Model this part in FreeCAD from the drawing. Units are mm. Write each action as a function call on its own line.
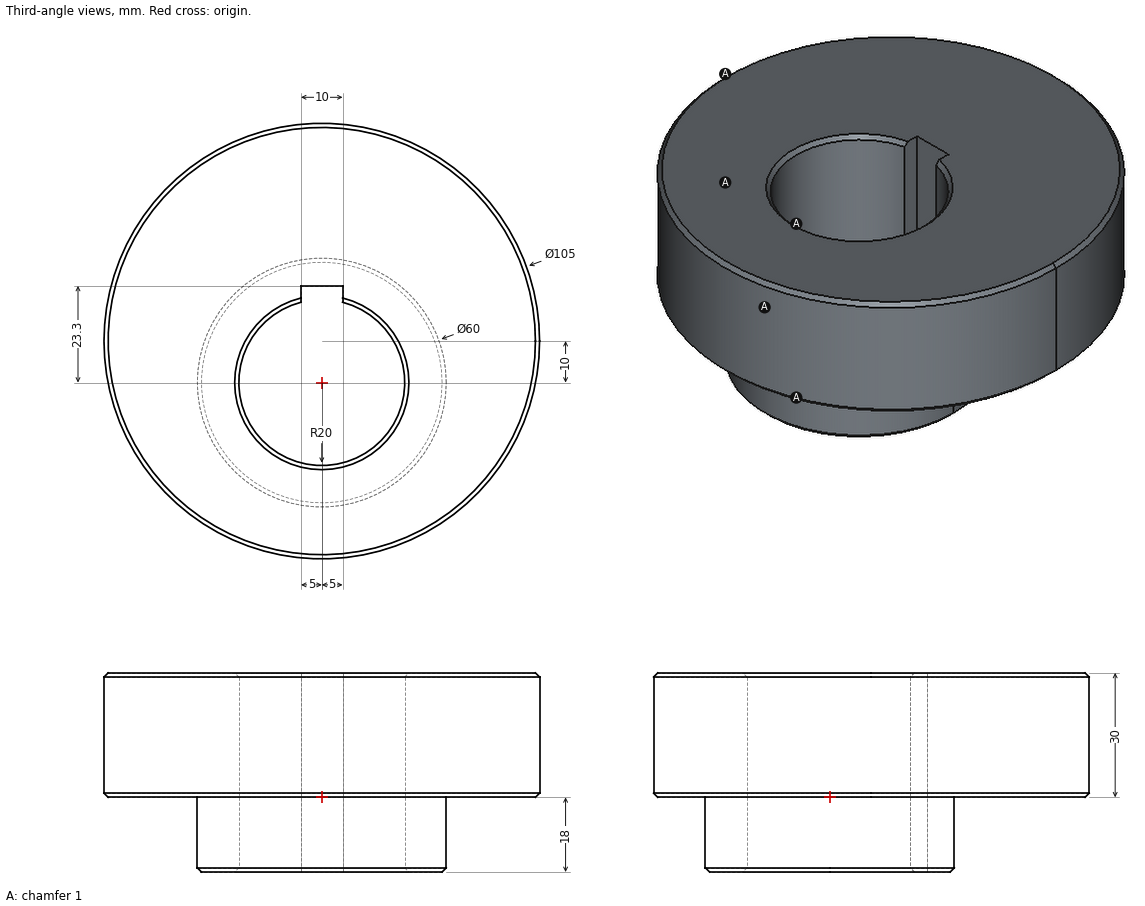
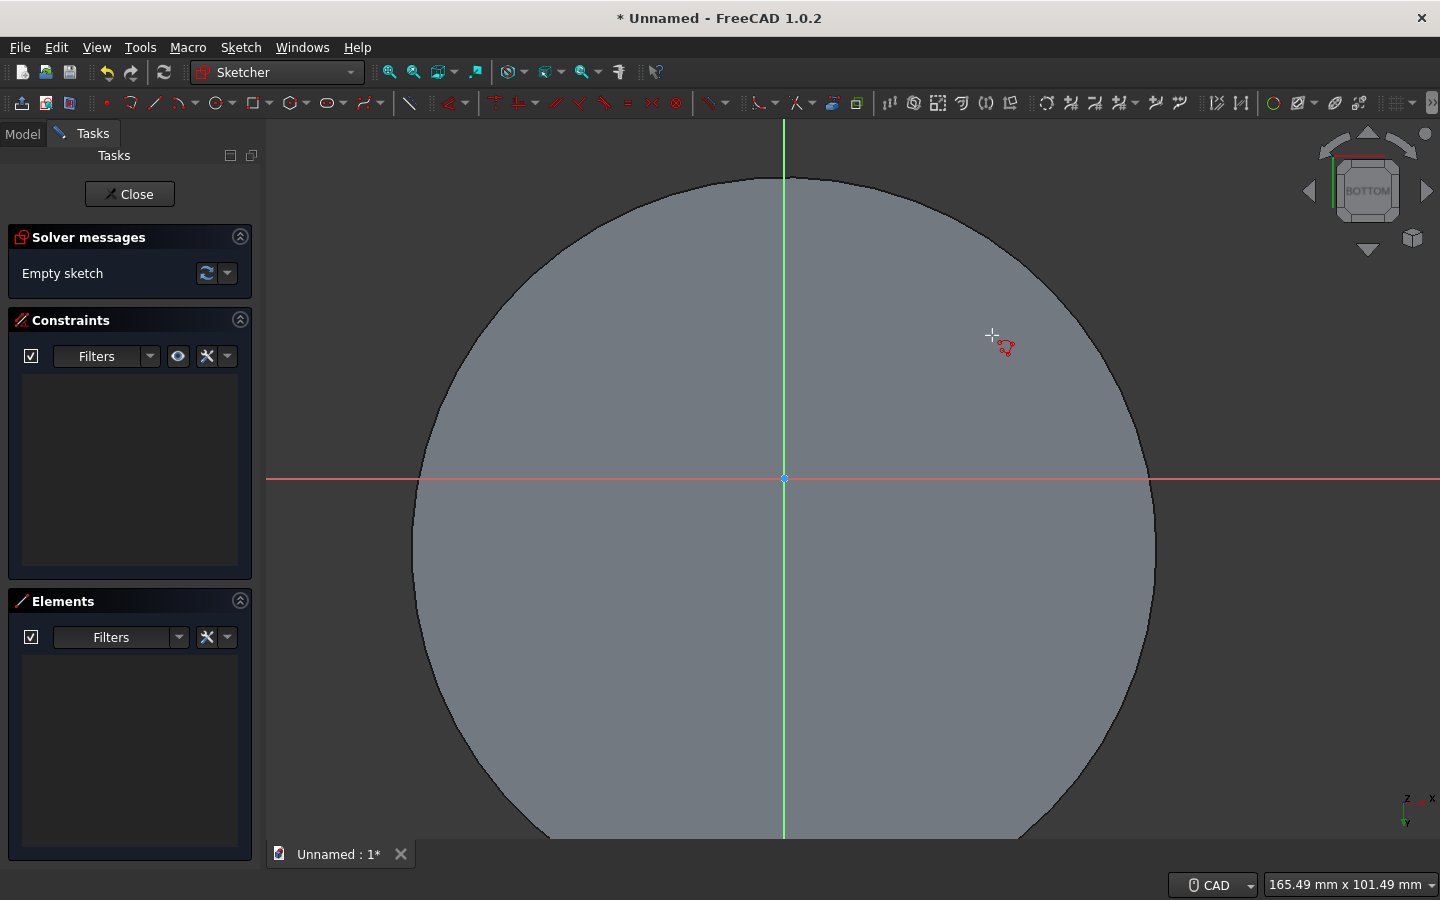
click(749, 616)
click(749, 644)
click(820, 644)
click(820, 616)
right_click(820, 616)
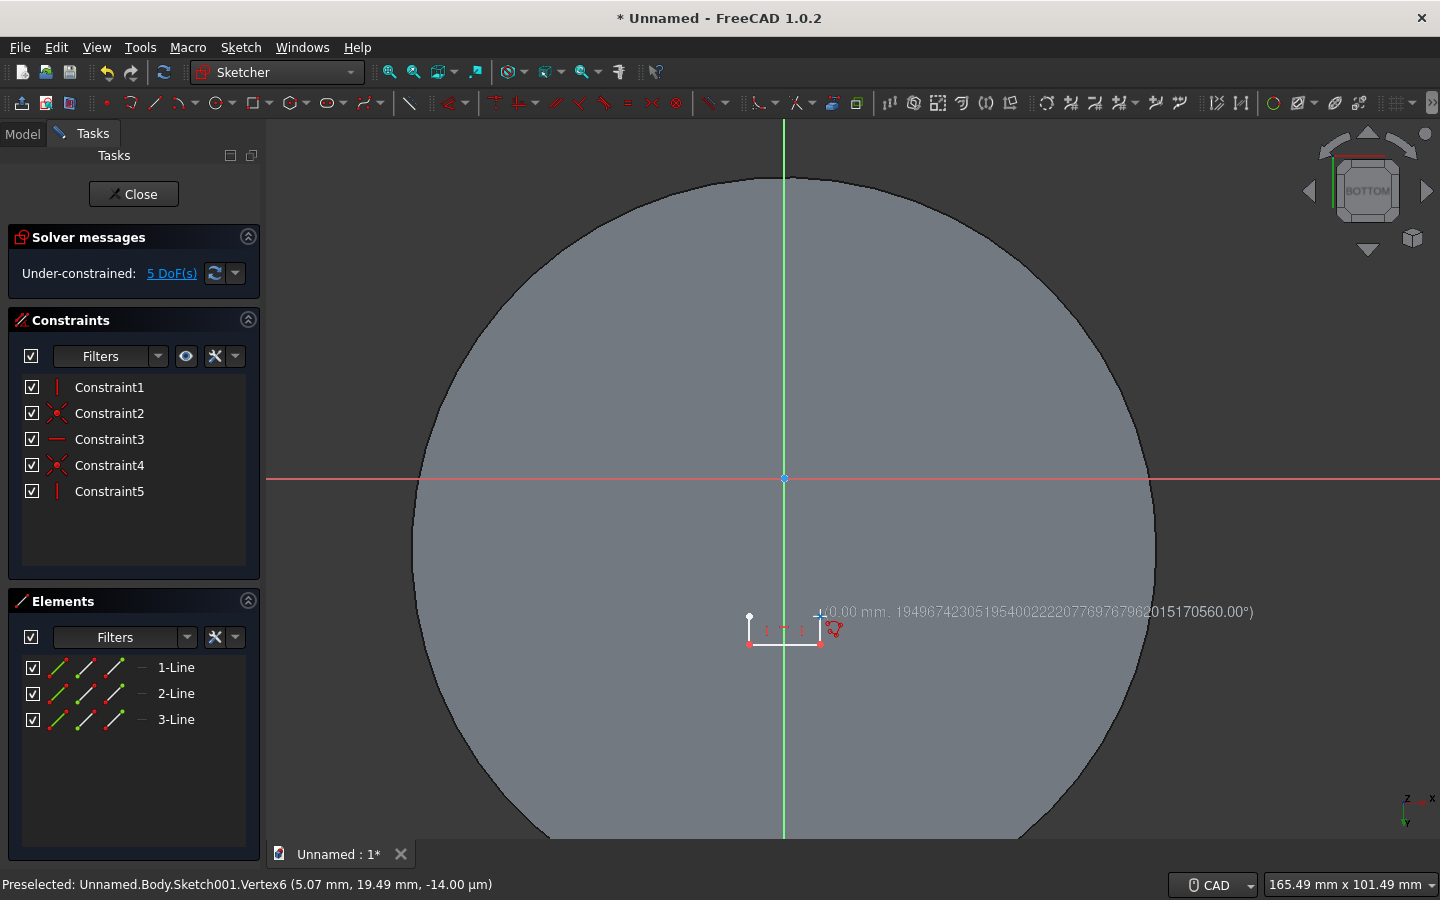
key(g)
key(3)
key(a)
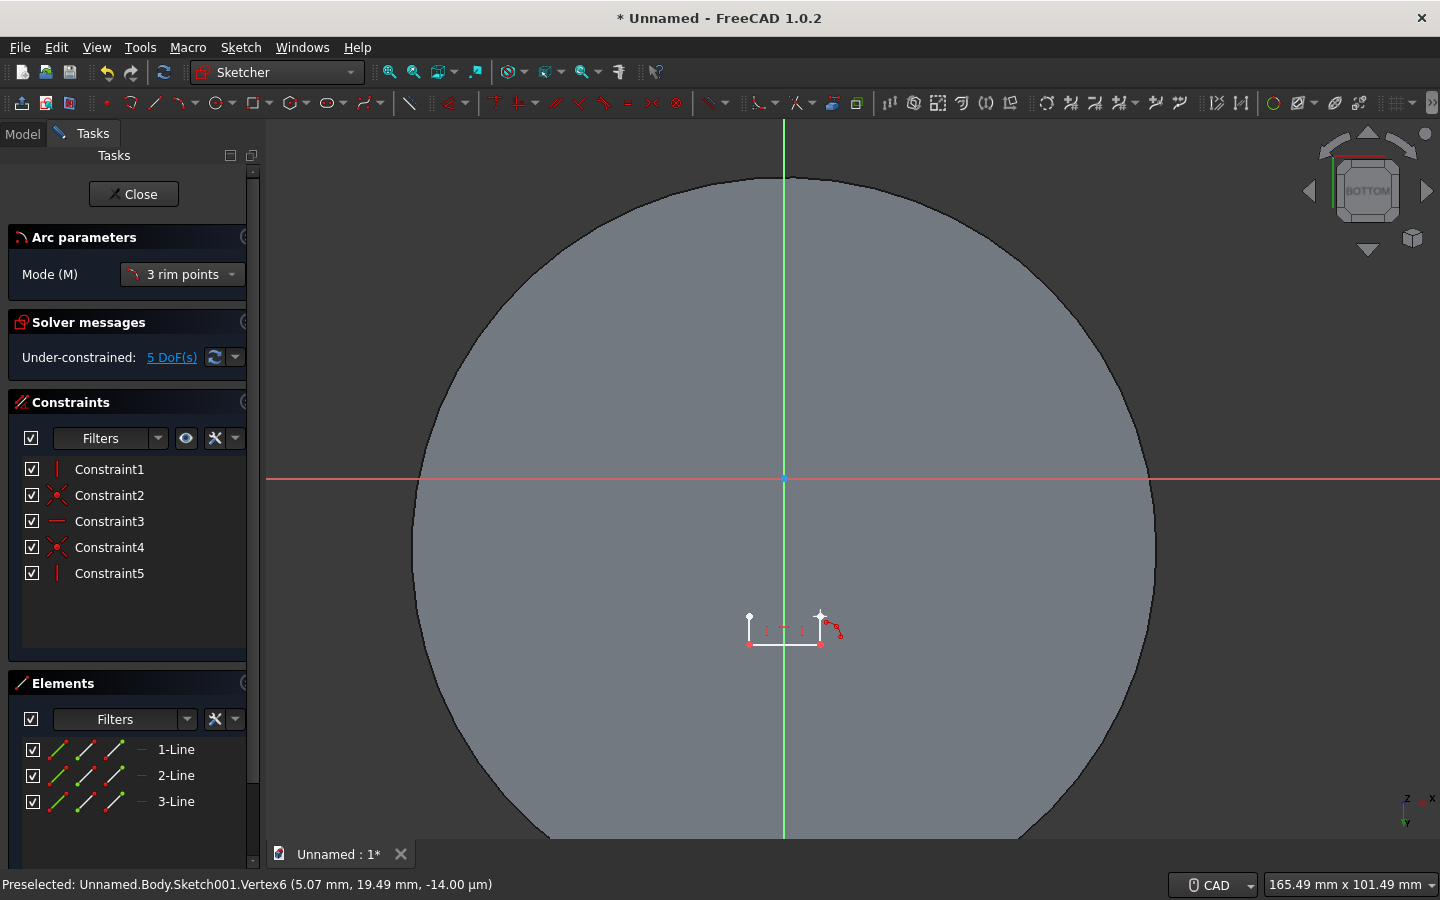
click(820, 617)
click(749, 617)
click(862, 360)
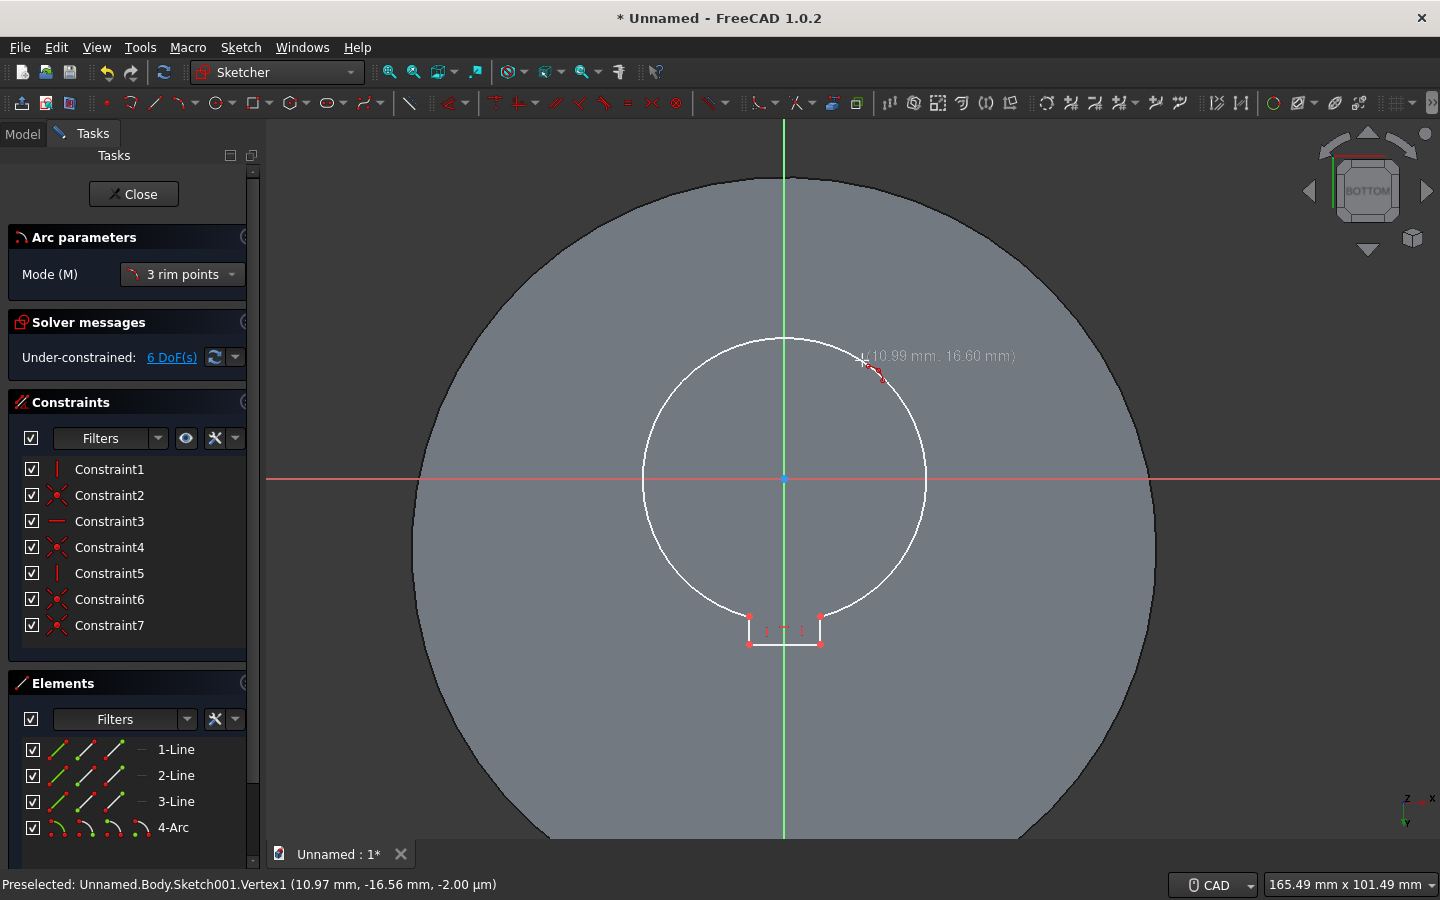
click(216, 104)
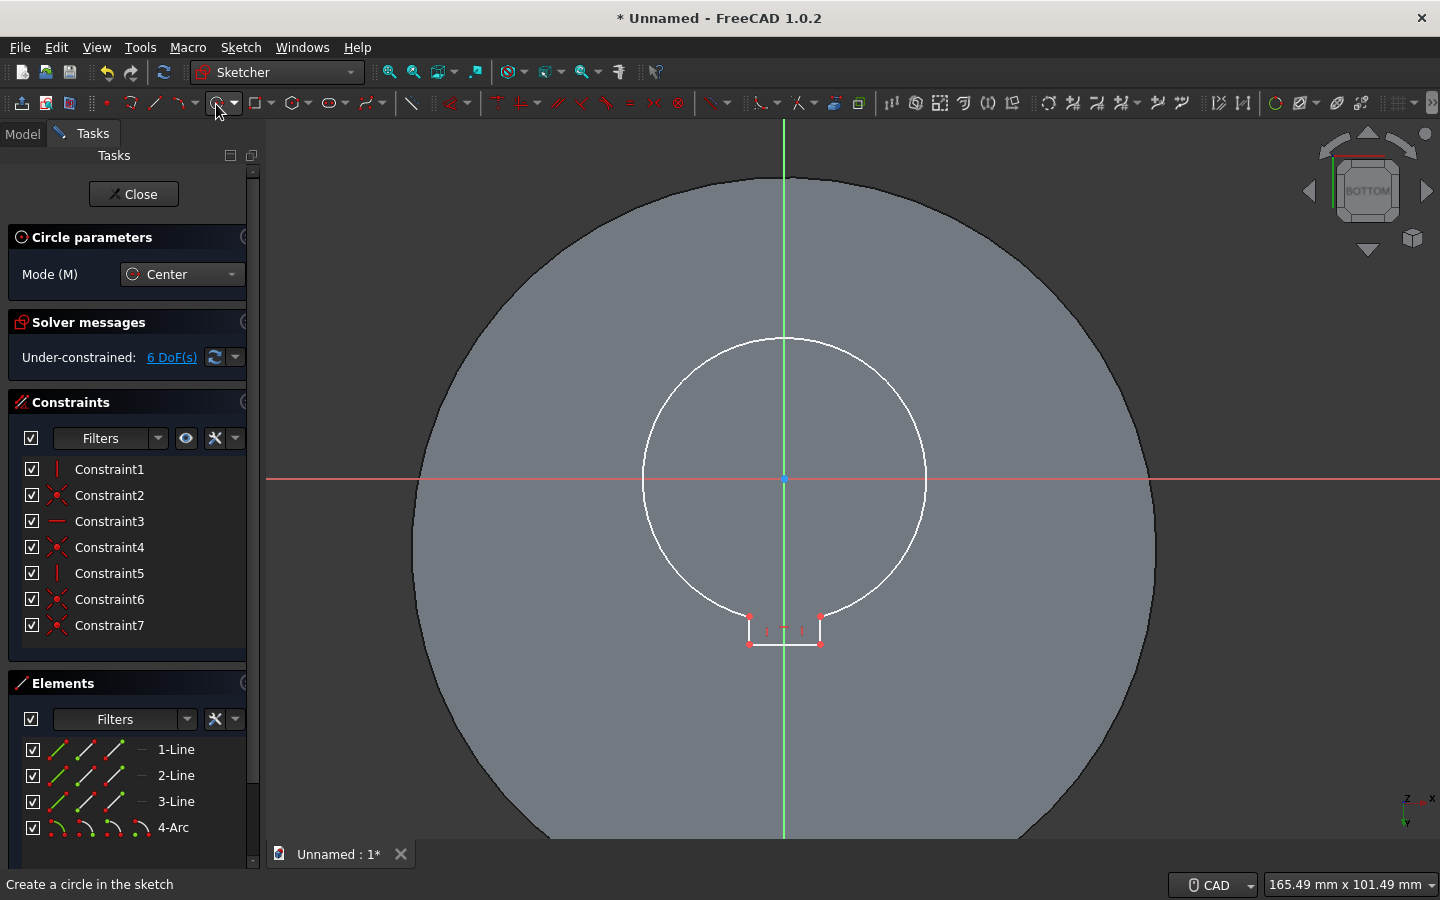
click(784, 479)
move(935, 328)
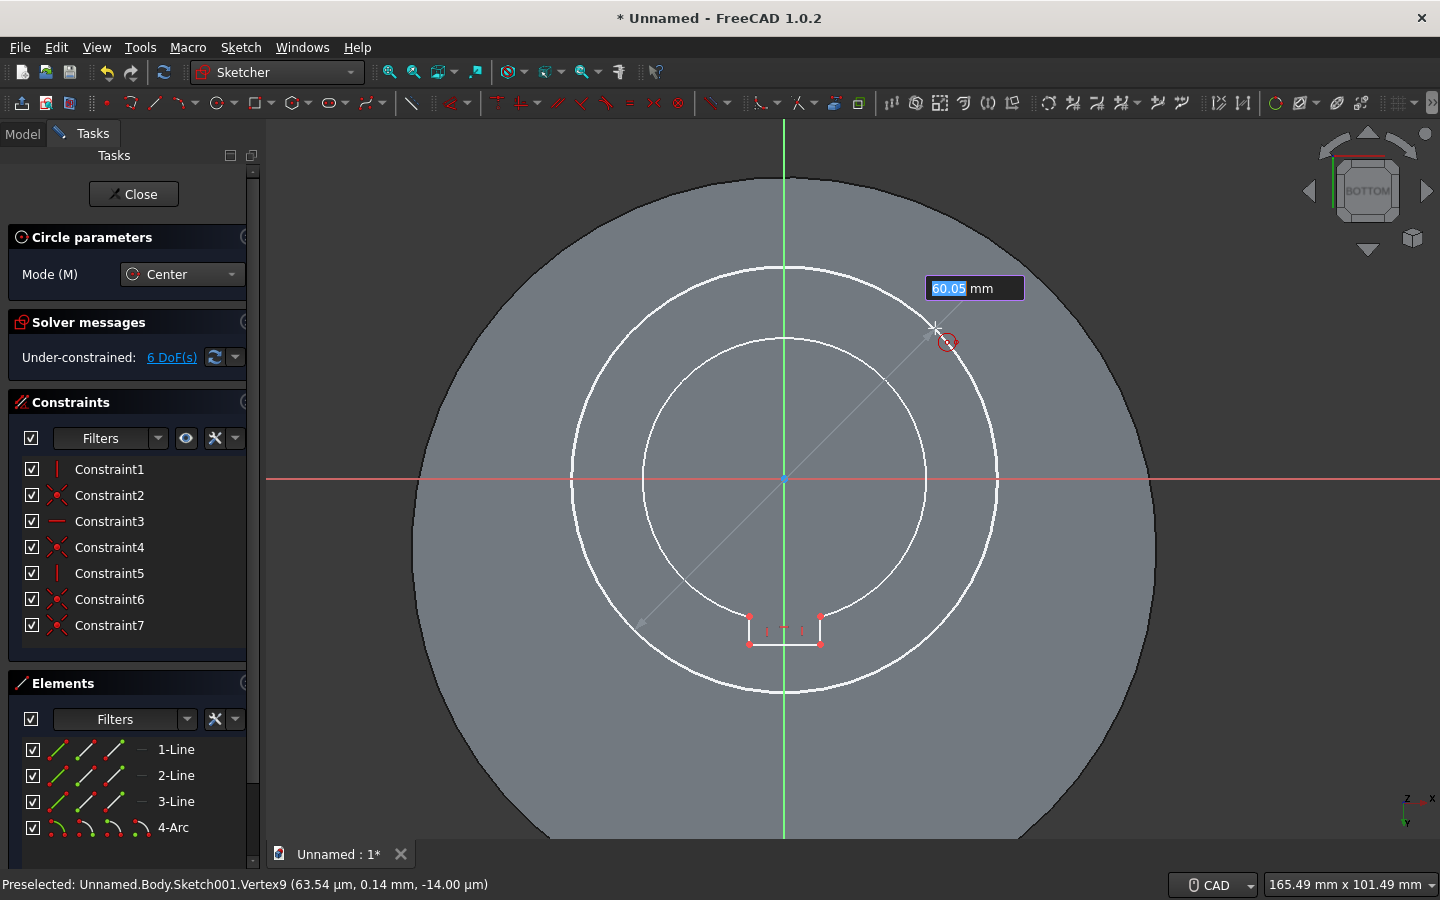
text(60)
key(Return)
key(Escape)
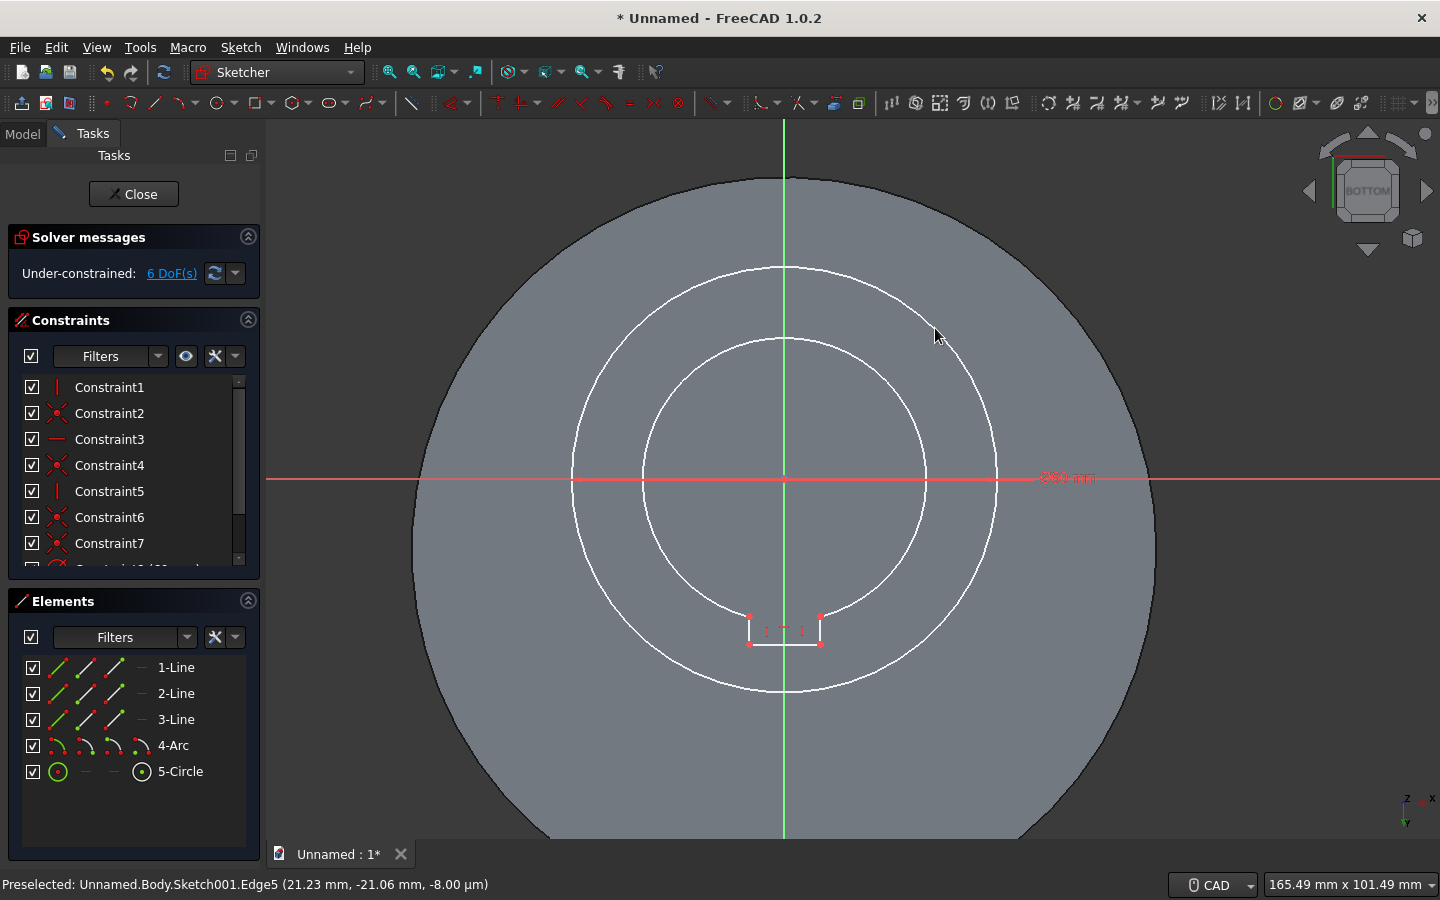
drag(774, 469, 794, 490)